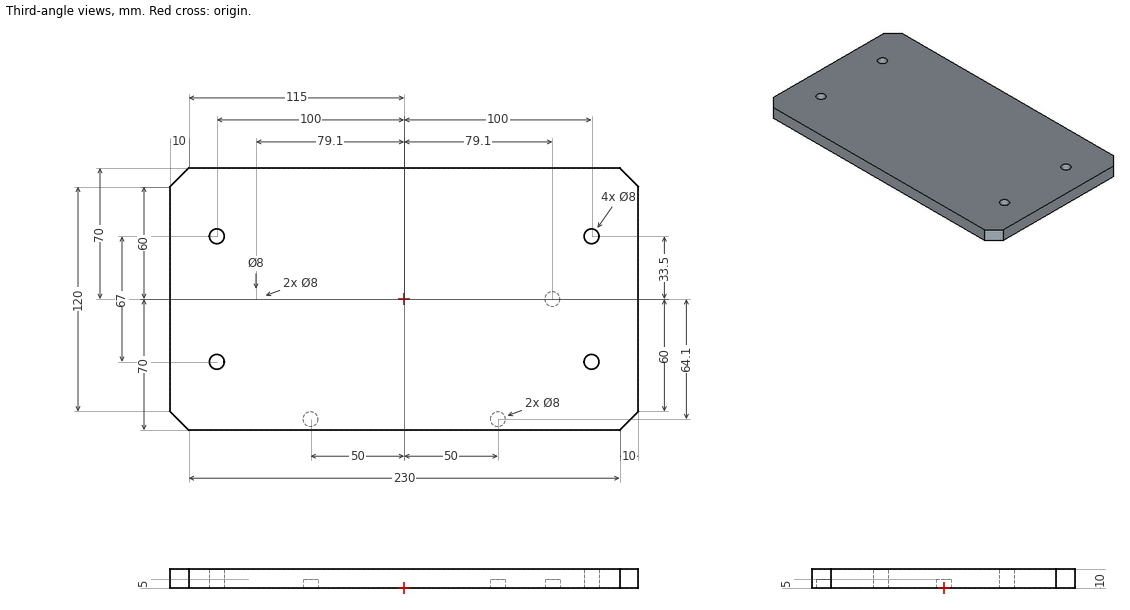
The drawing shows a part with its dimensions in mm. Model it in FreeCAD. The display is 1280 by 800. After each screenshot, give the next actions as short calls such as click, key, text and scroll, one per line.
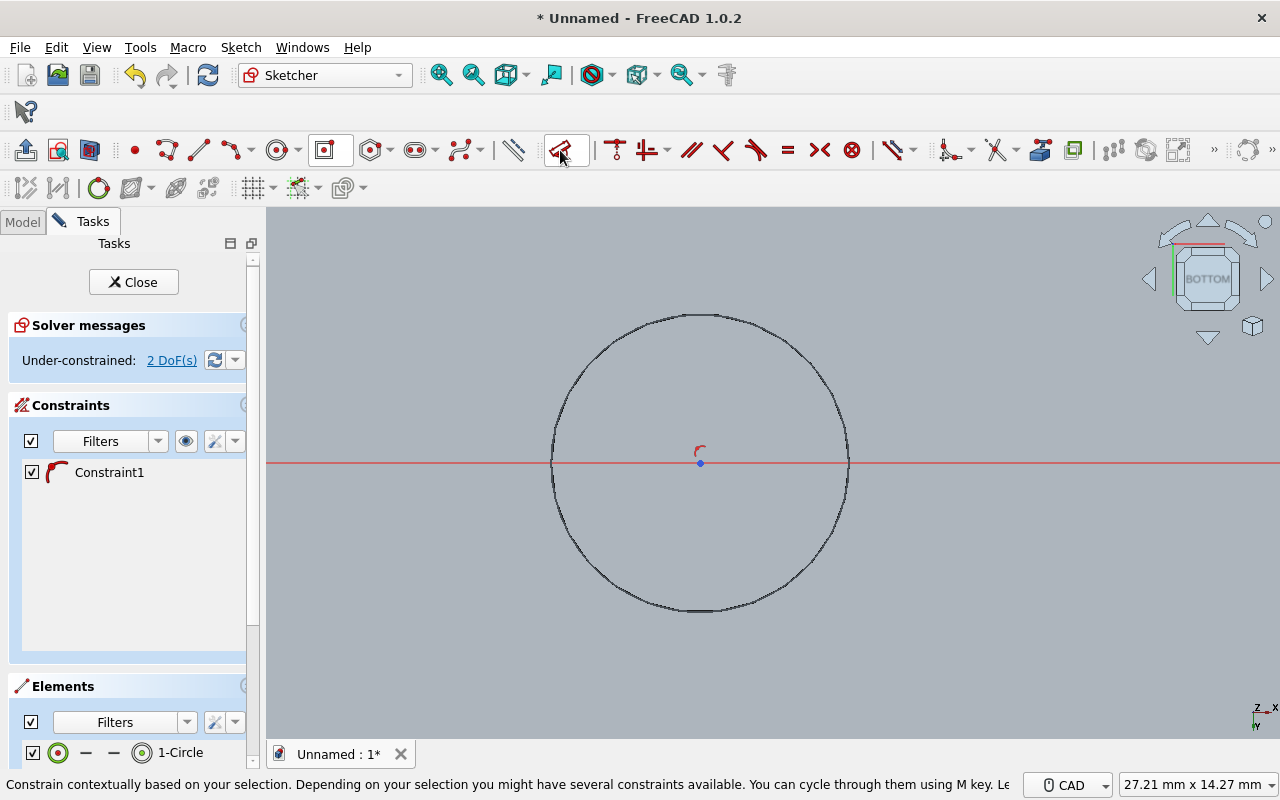
click(805, 358)
click(828, 335)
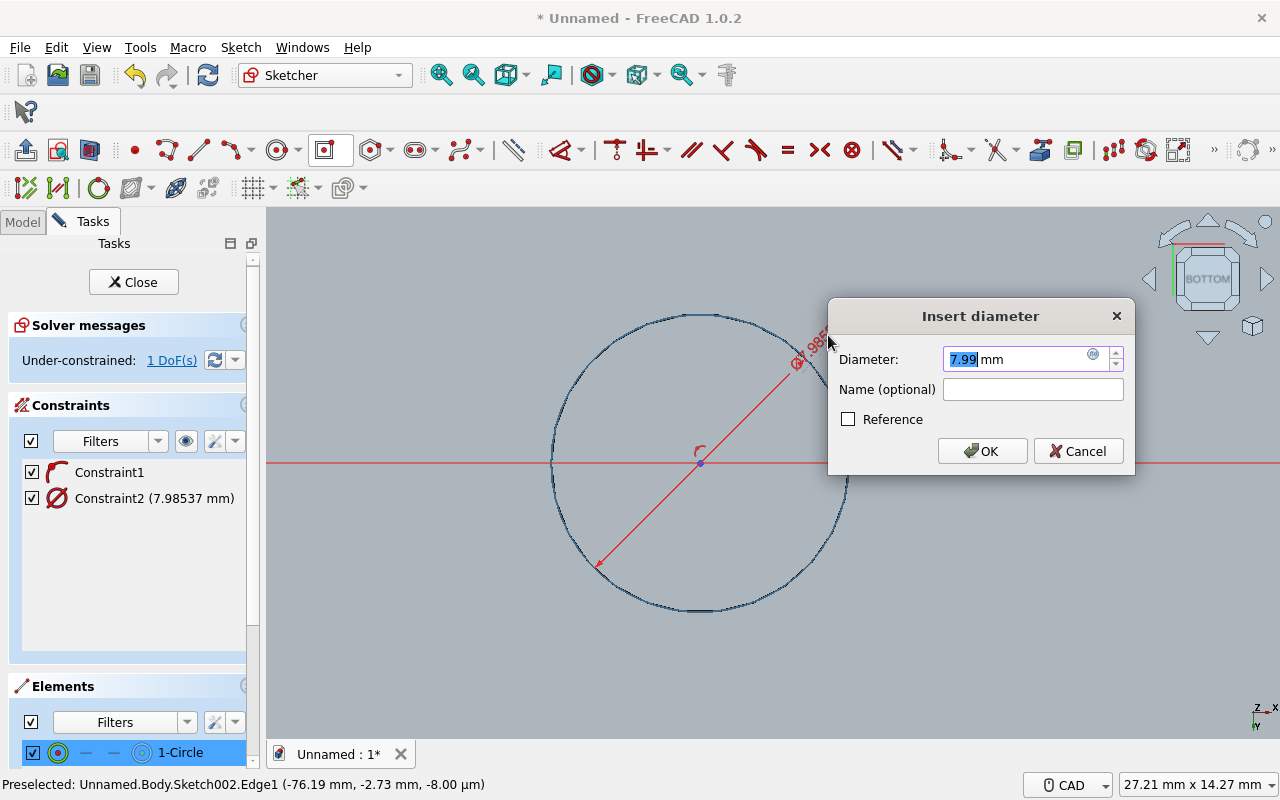
text(8)
key(Return)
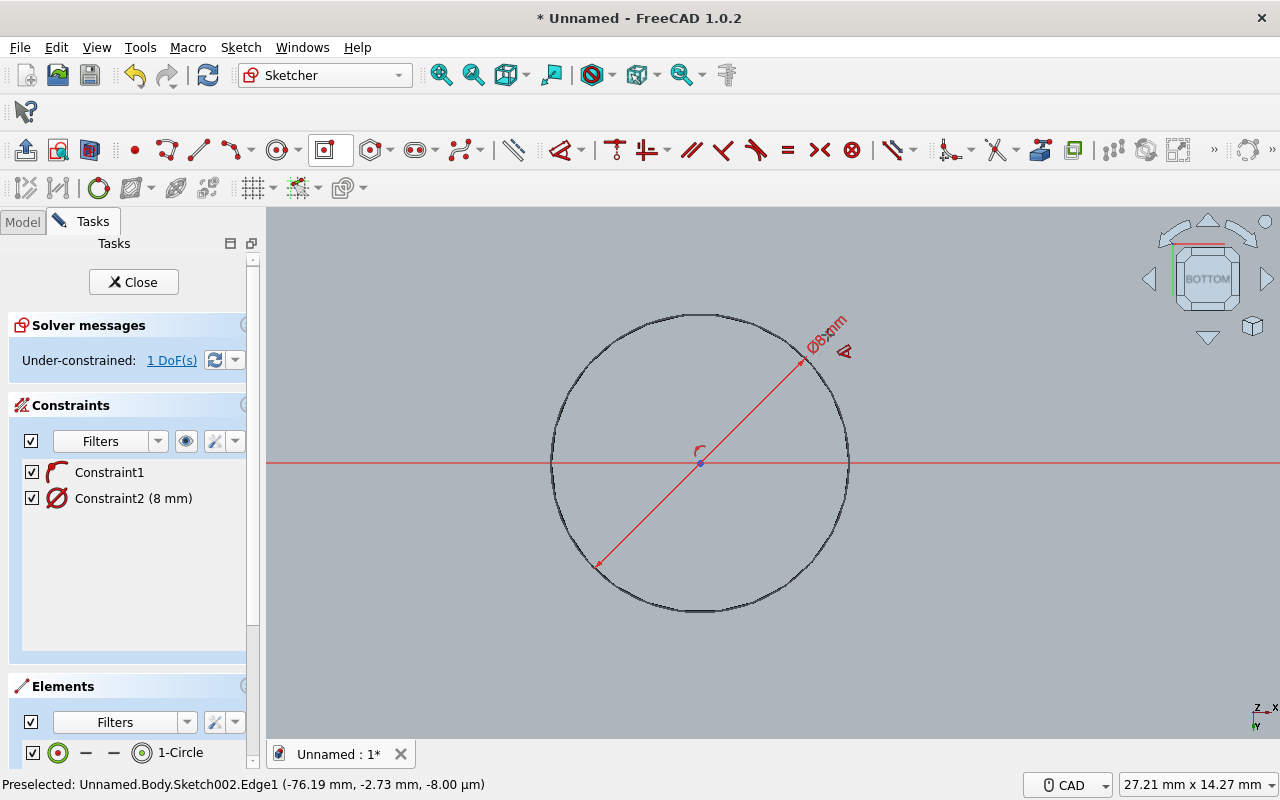
click(700, 463)
click(908, 497)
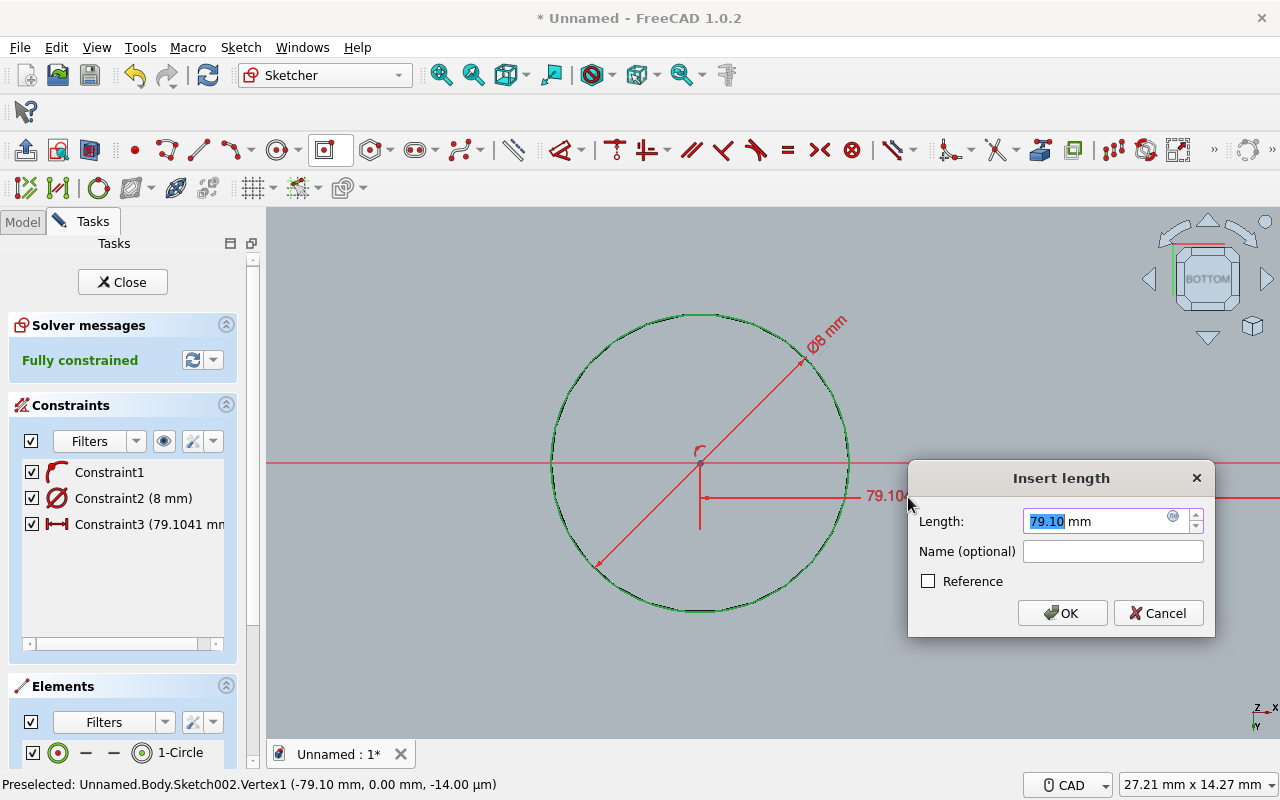
text(79.1)
key(Return)
key(Escape)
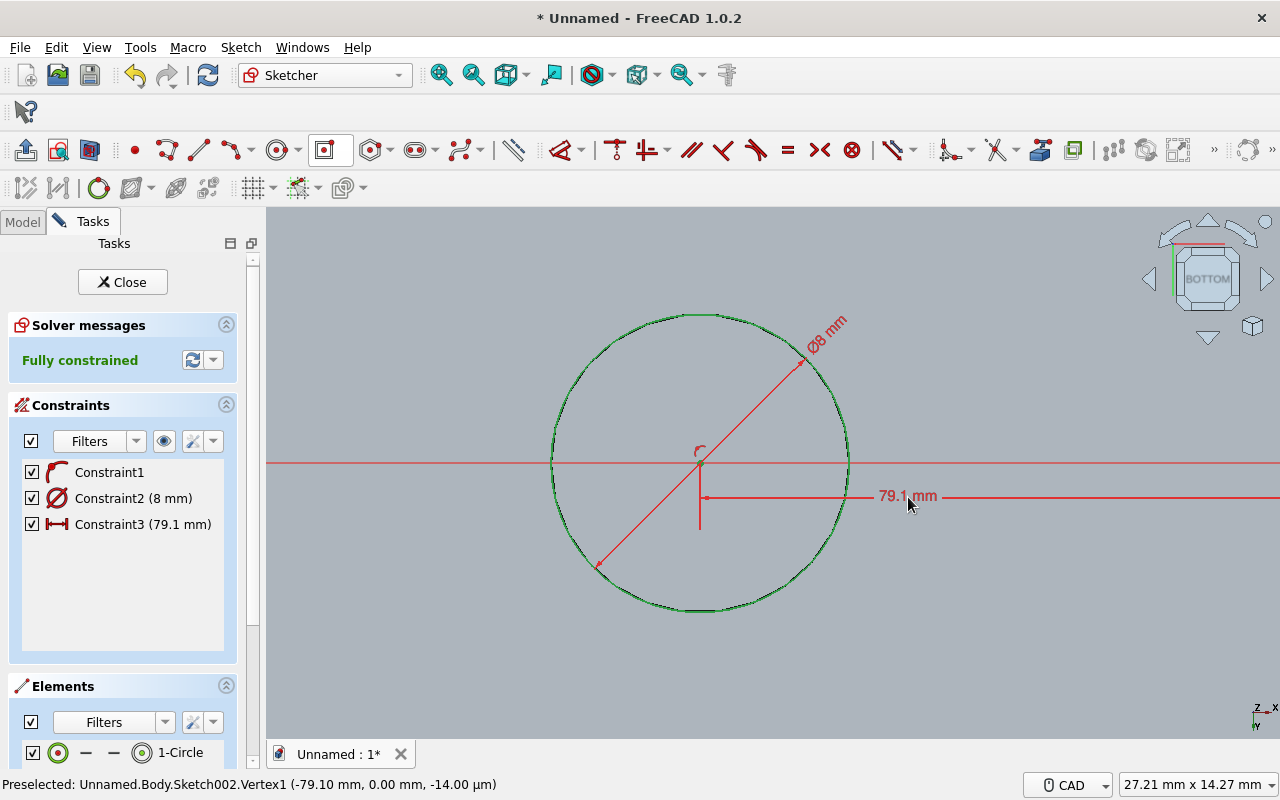
click(123, 282)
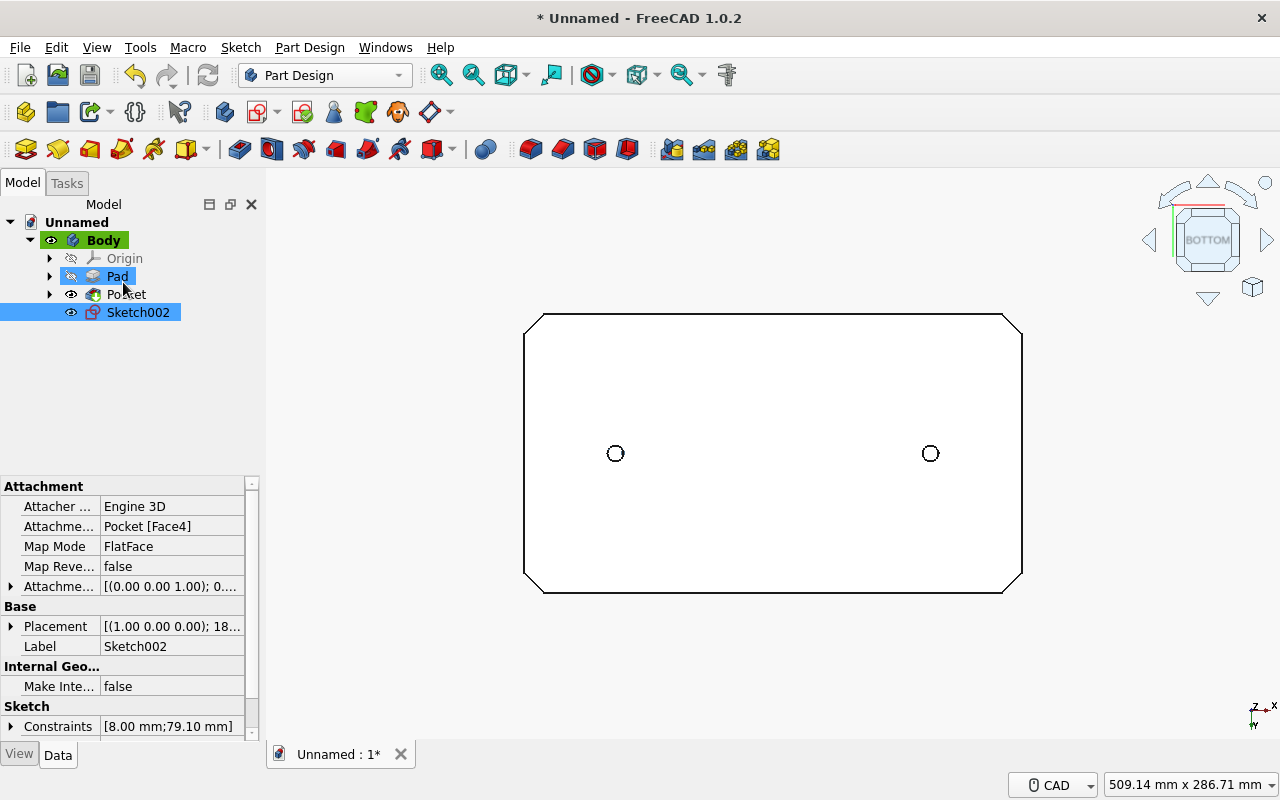
click(26, 150)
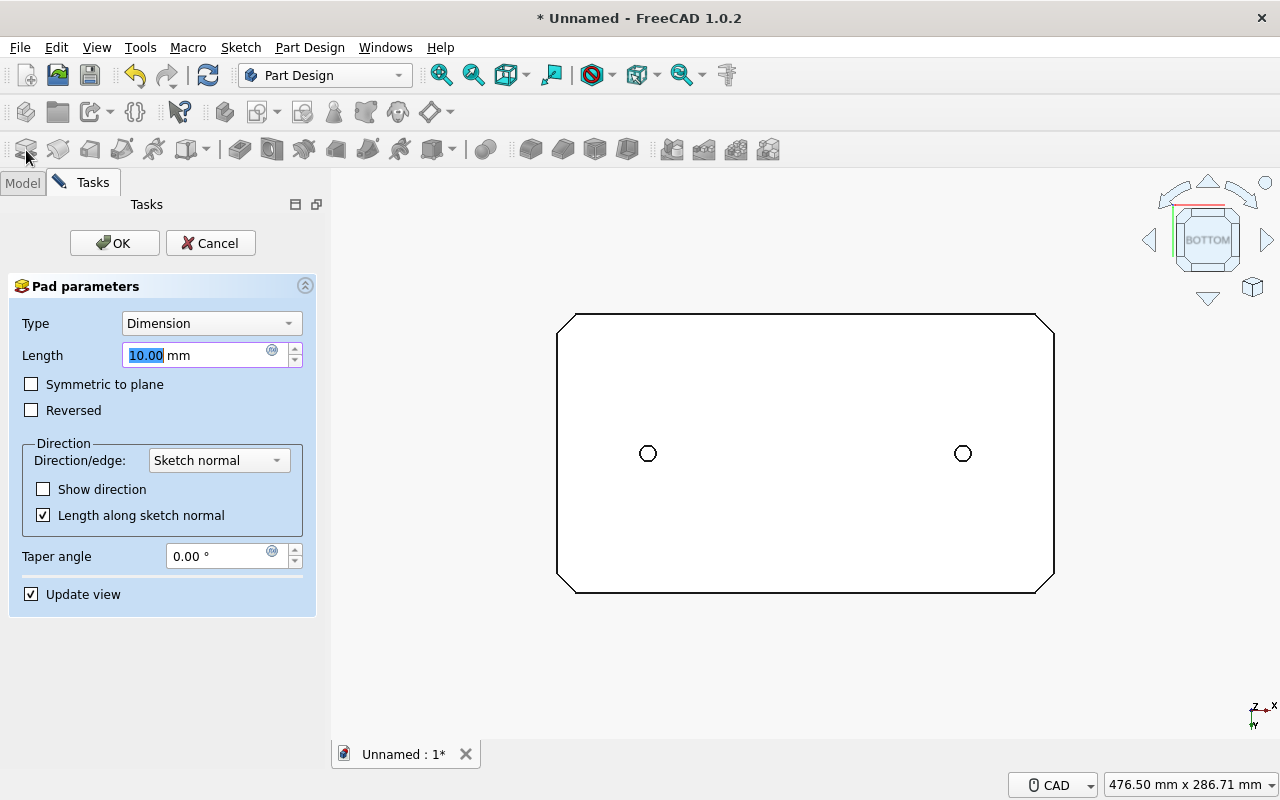
text(5)
key(Tab)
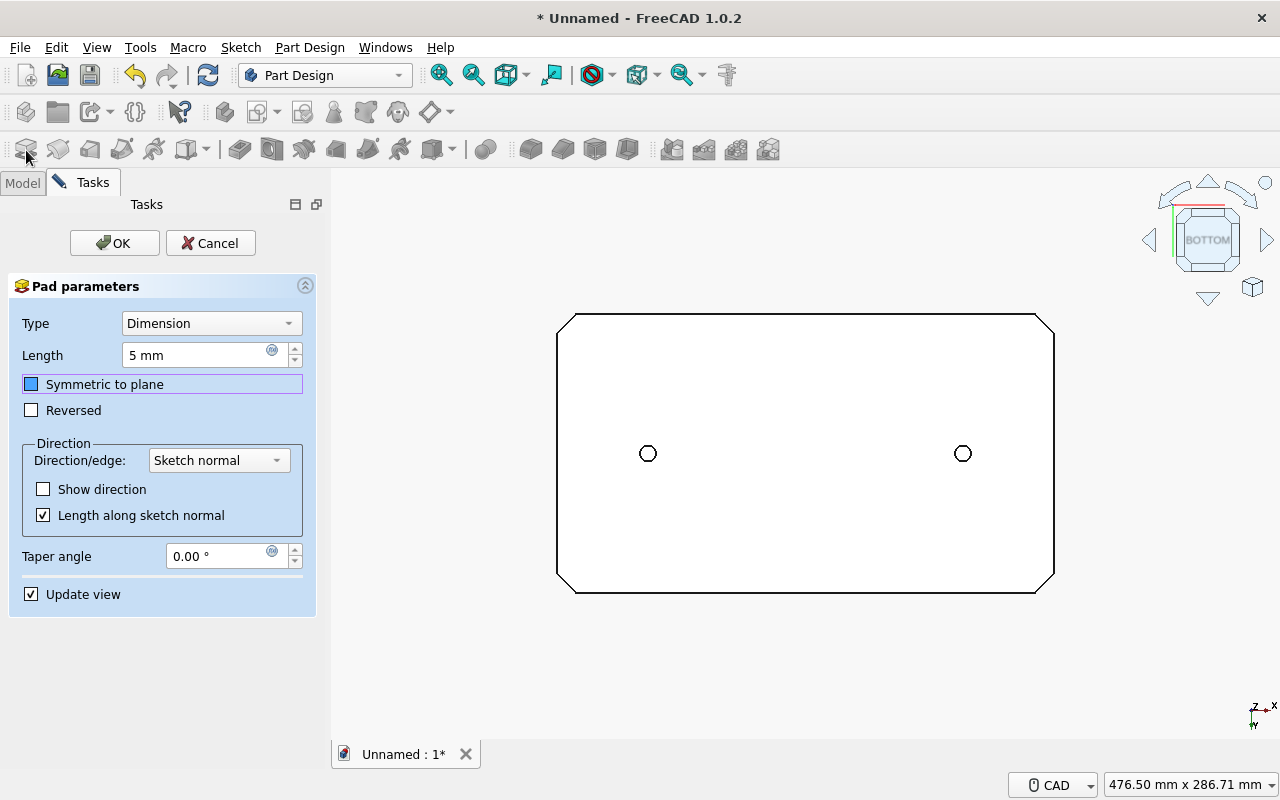
click(30, 410)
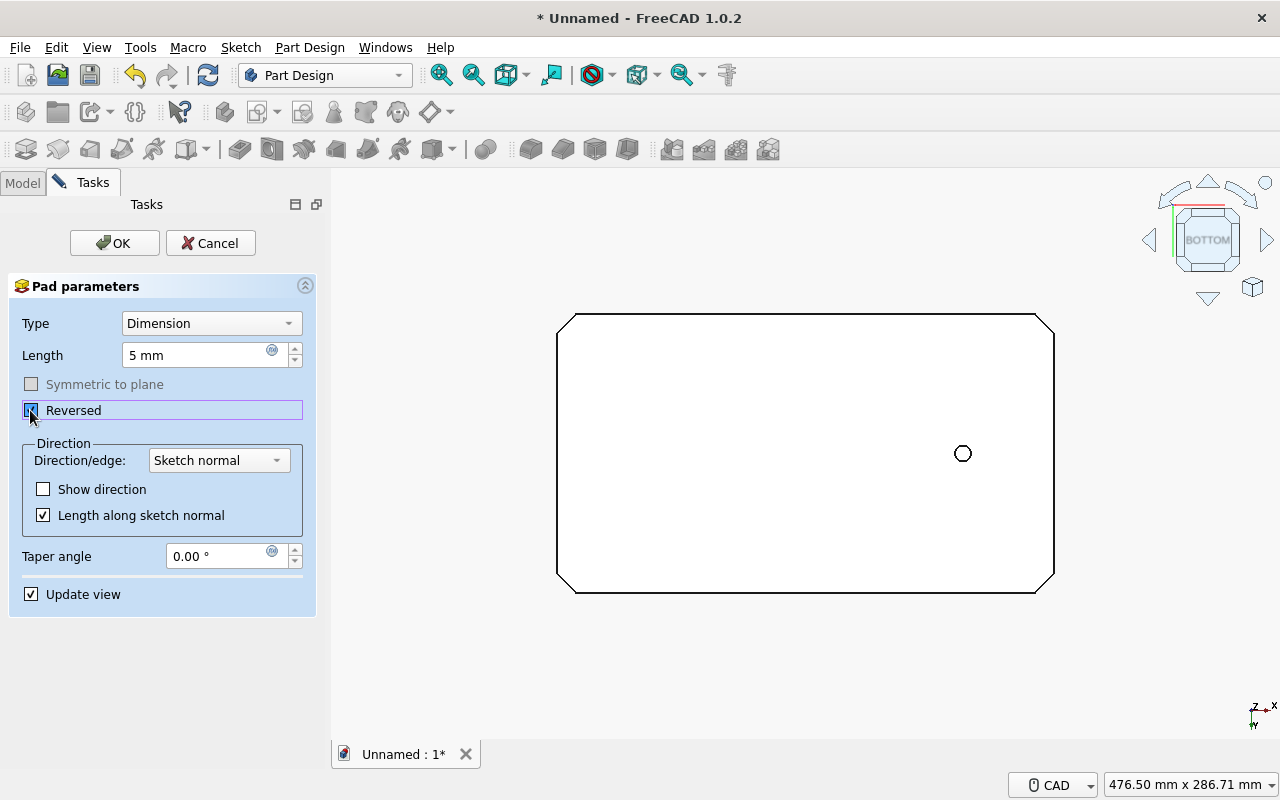
click(115, 243)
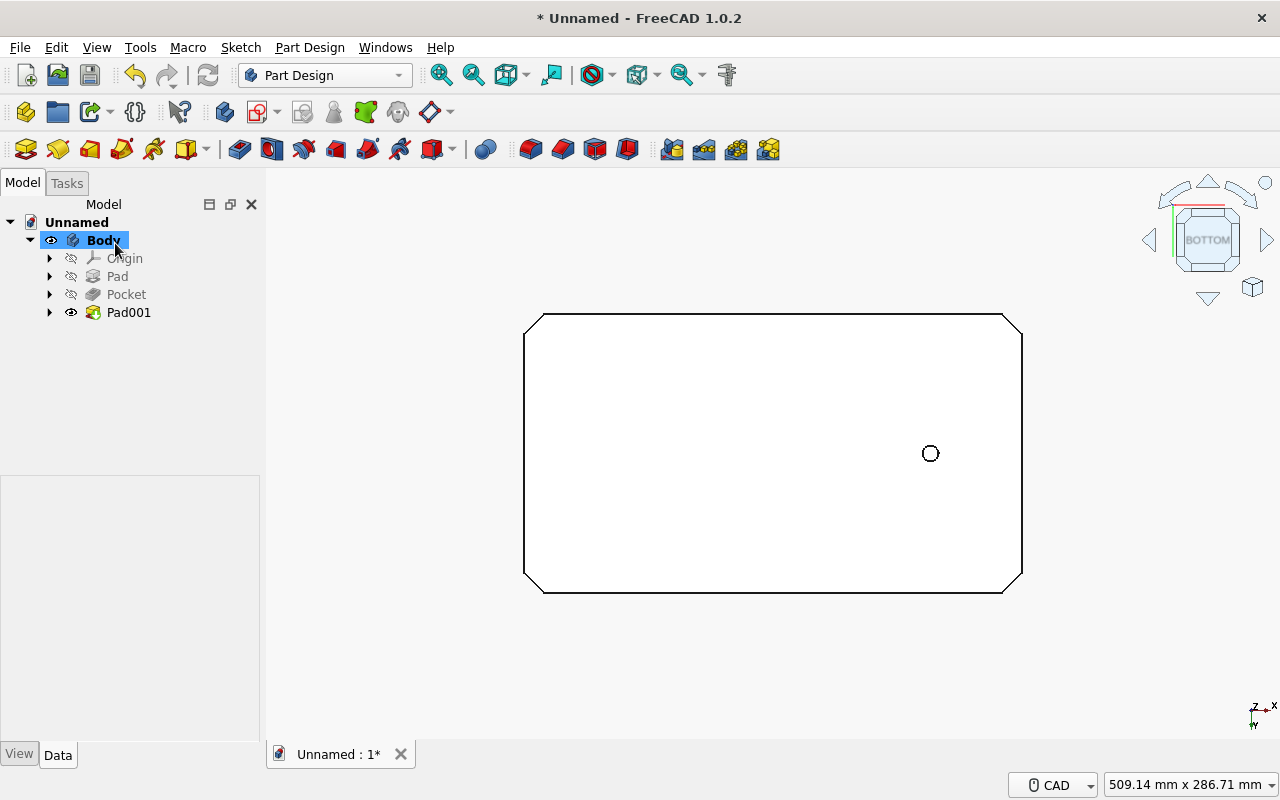
click(773, 453)